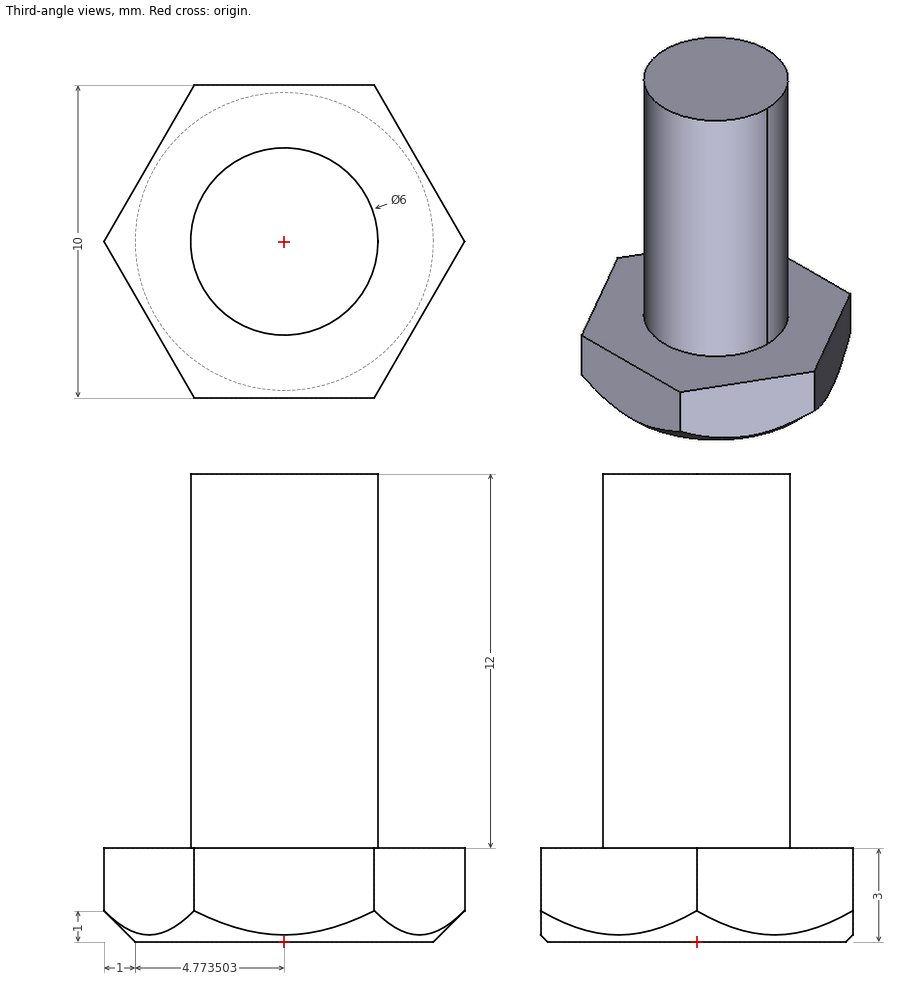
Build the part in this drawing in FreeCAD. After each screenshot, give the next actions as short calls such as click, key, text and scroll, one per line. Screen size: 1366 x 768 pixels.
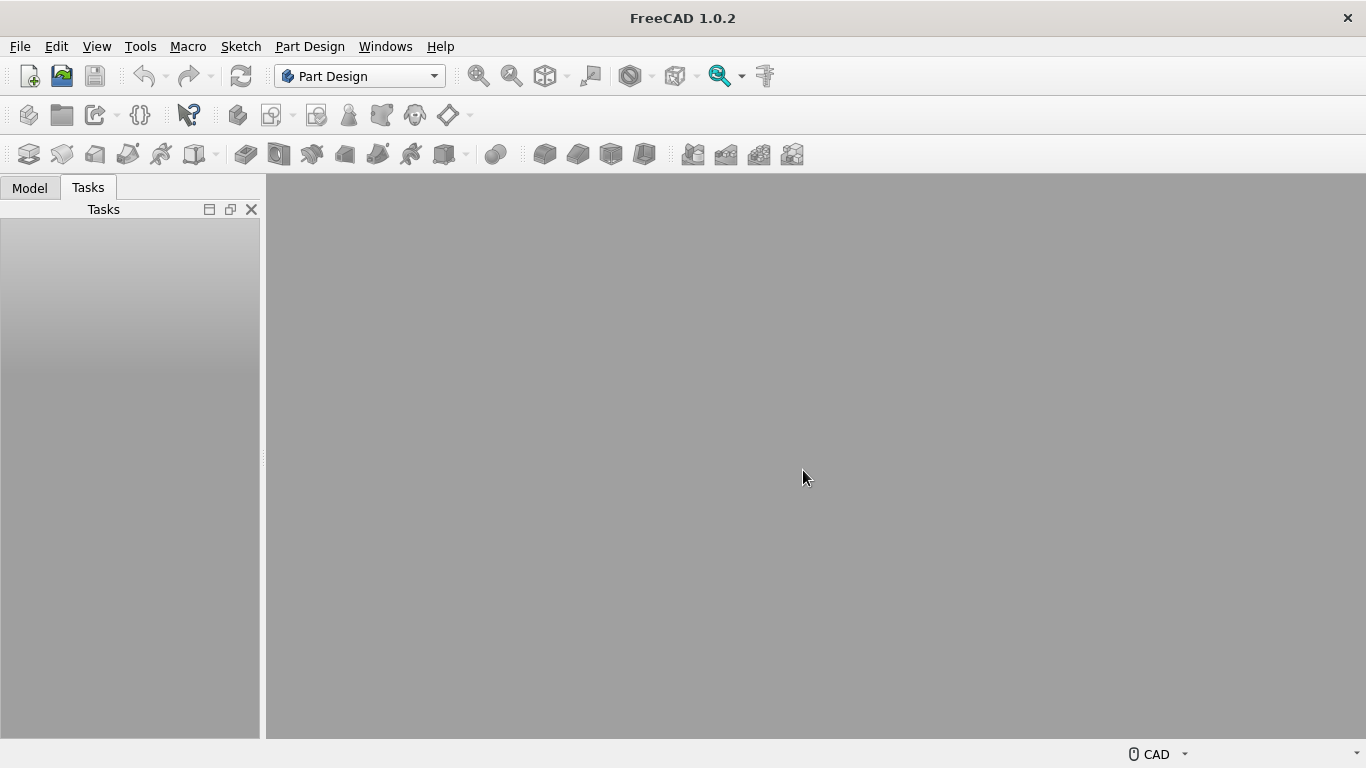
click(29, 76)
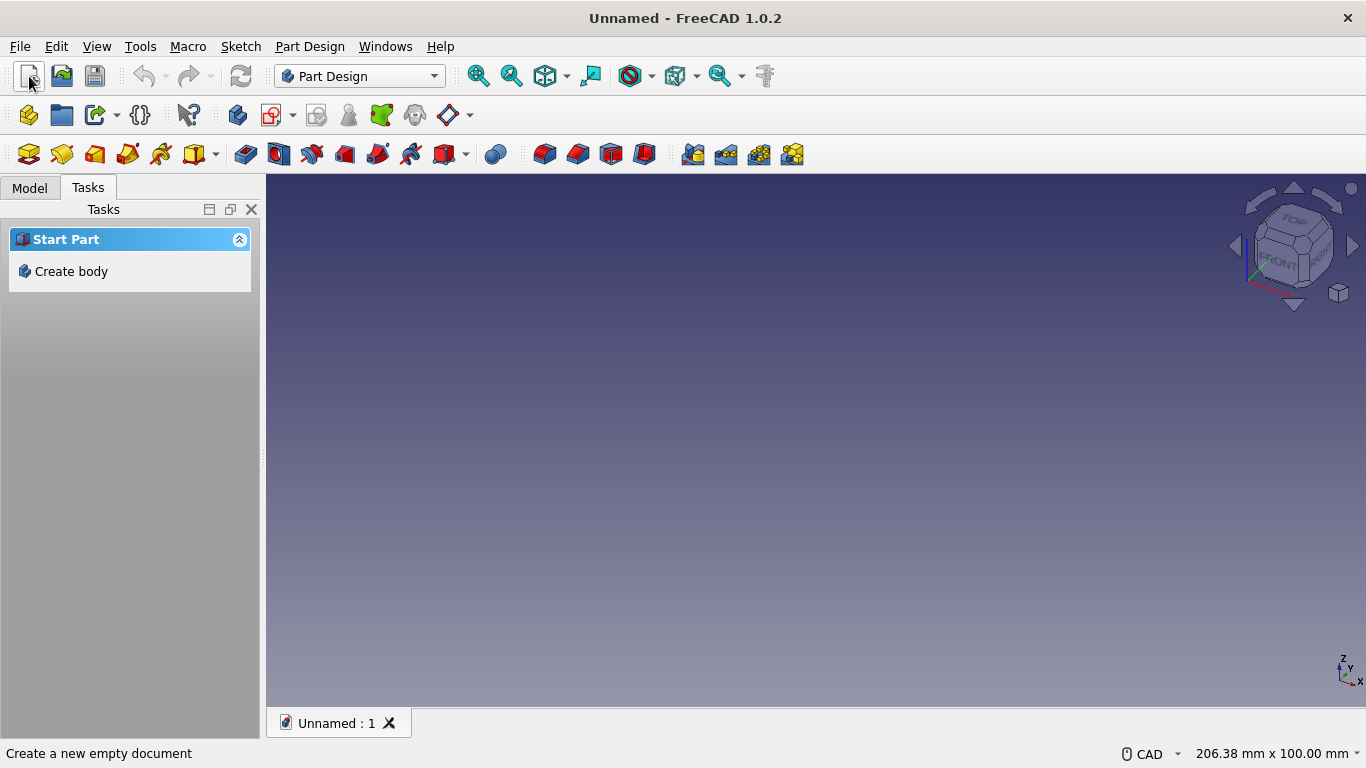
click(270, 116)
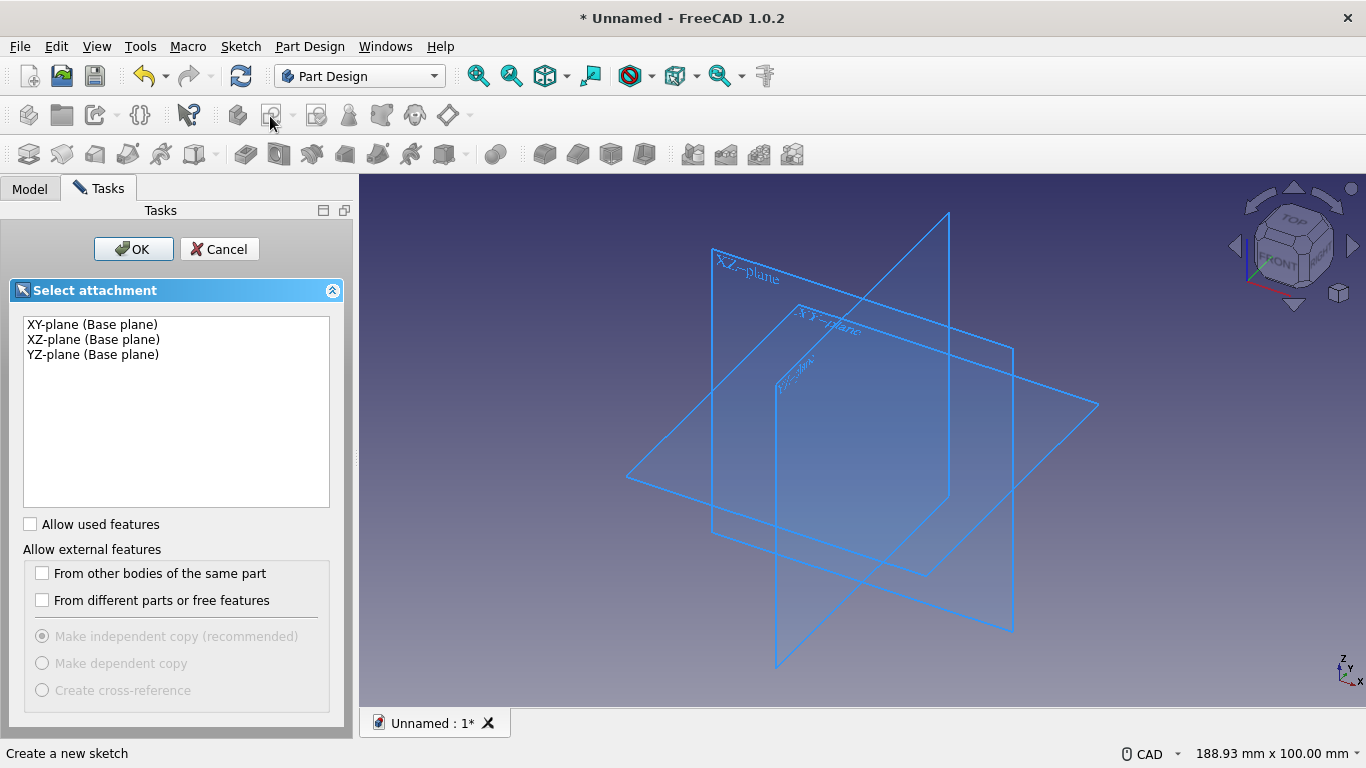
click(84, 324)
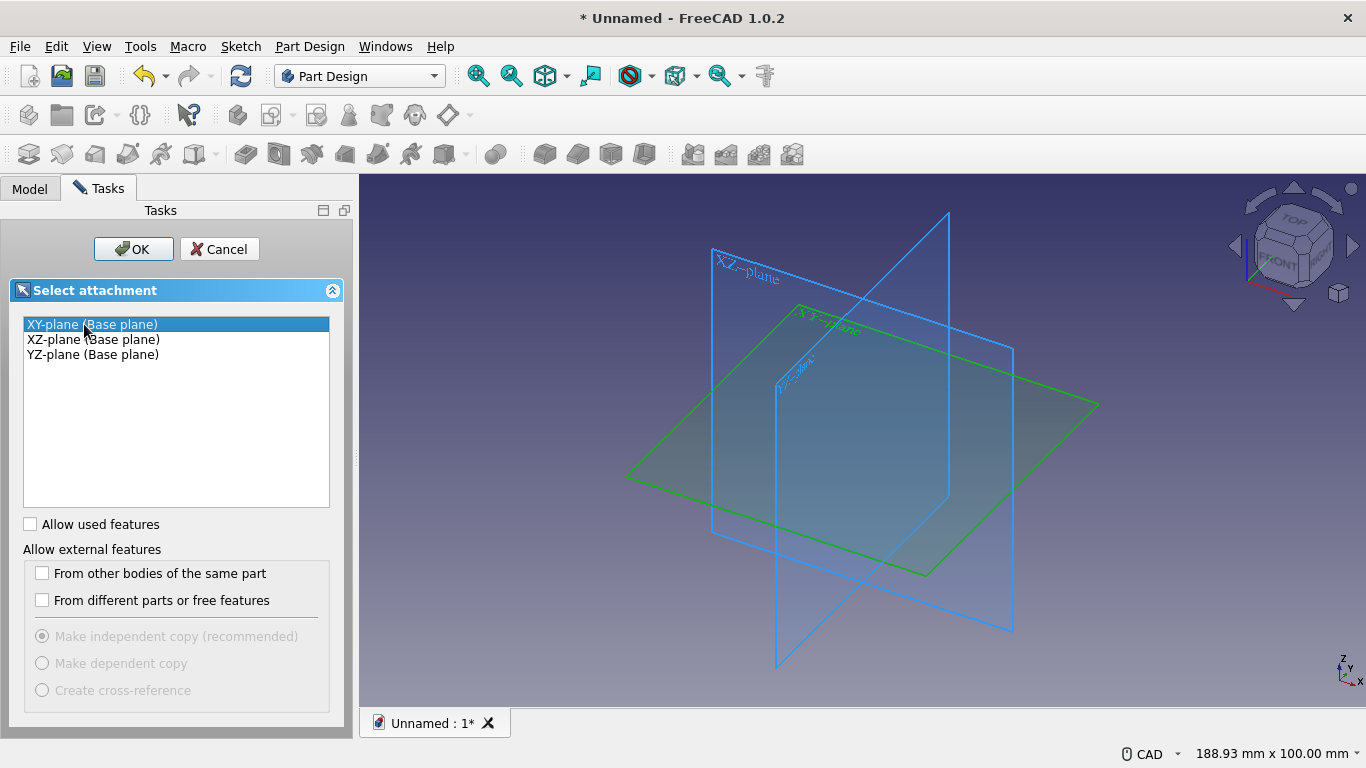
click(134, 249)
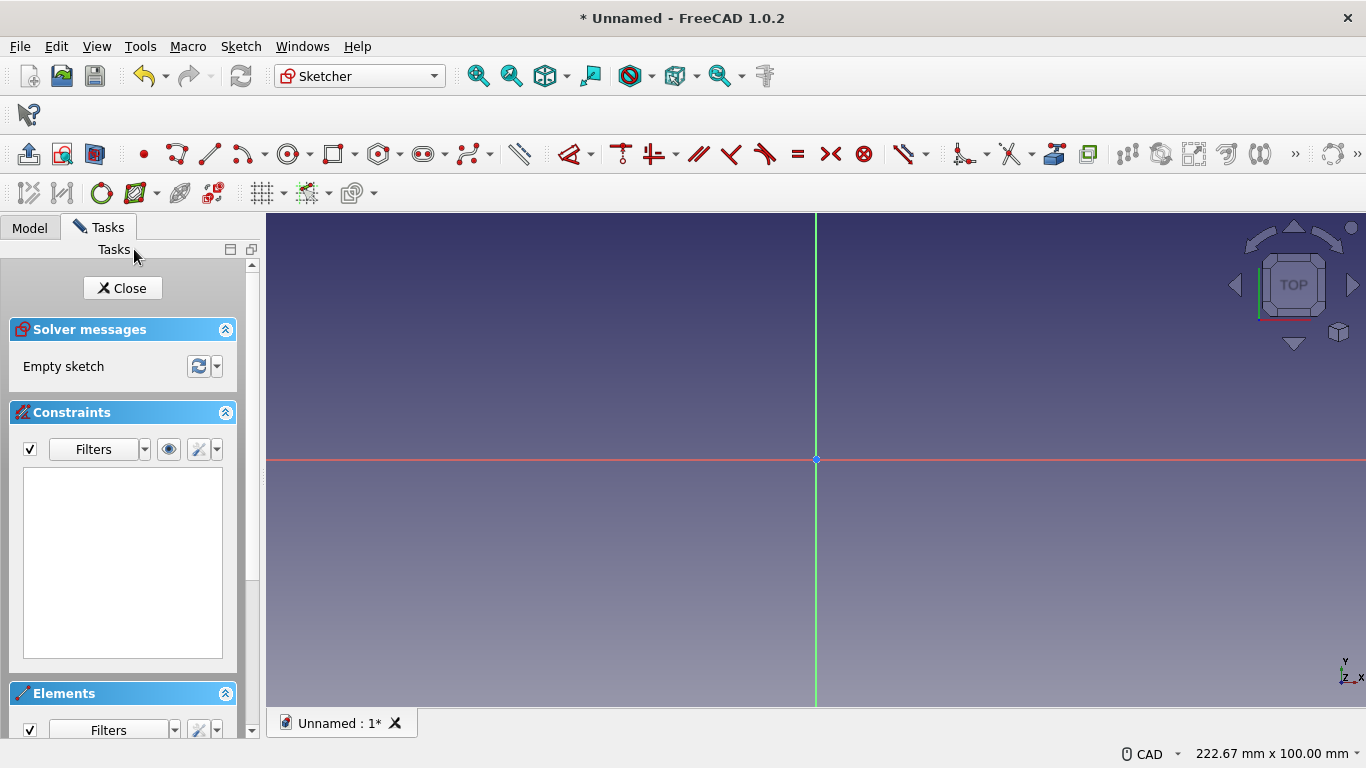
scroll(830, 460, up, 9)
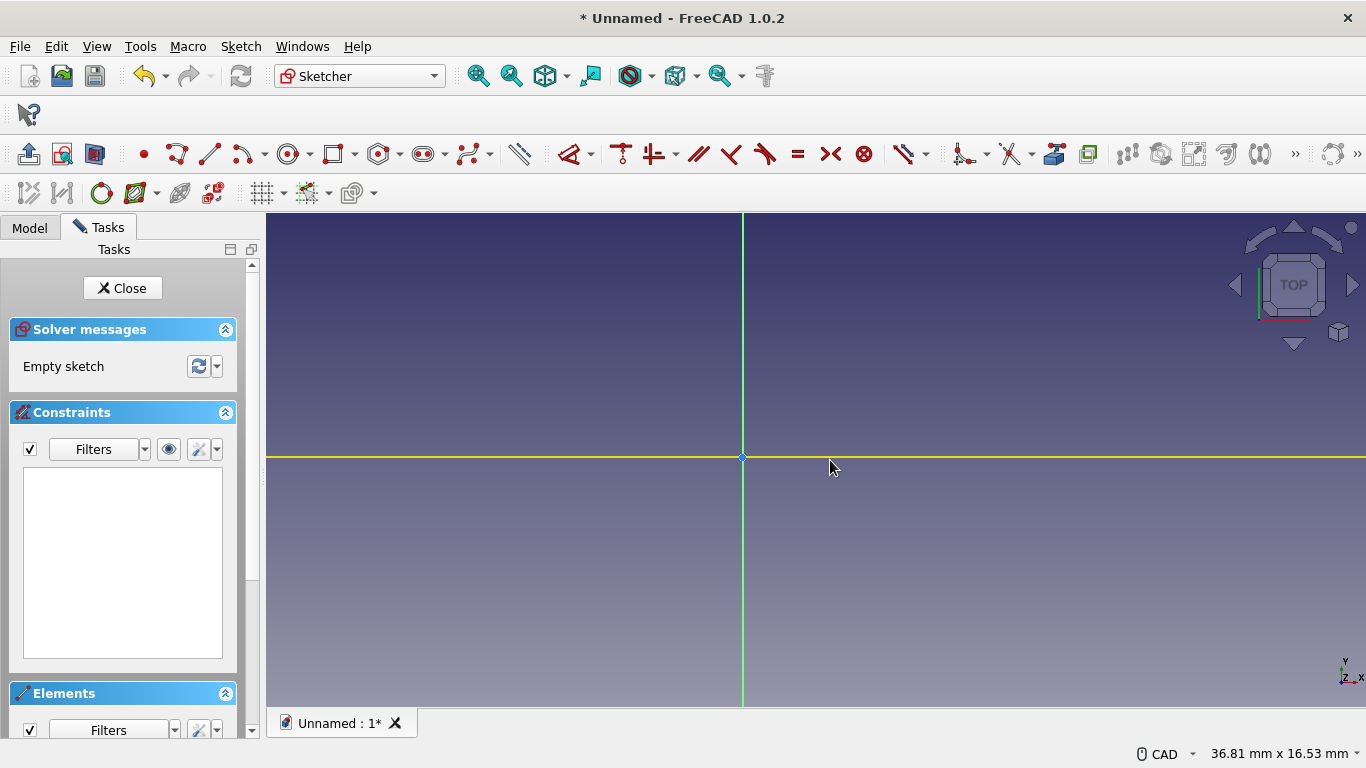
click(378, 154)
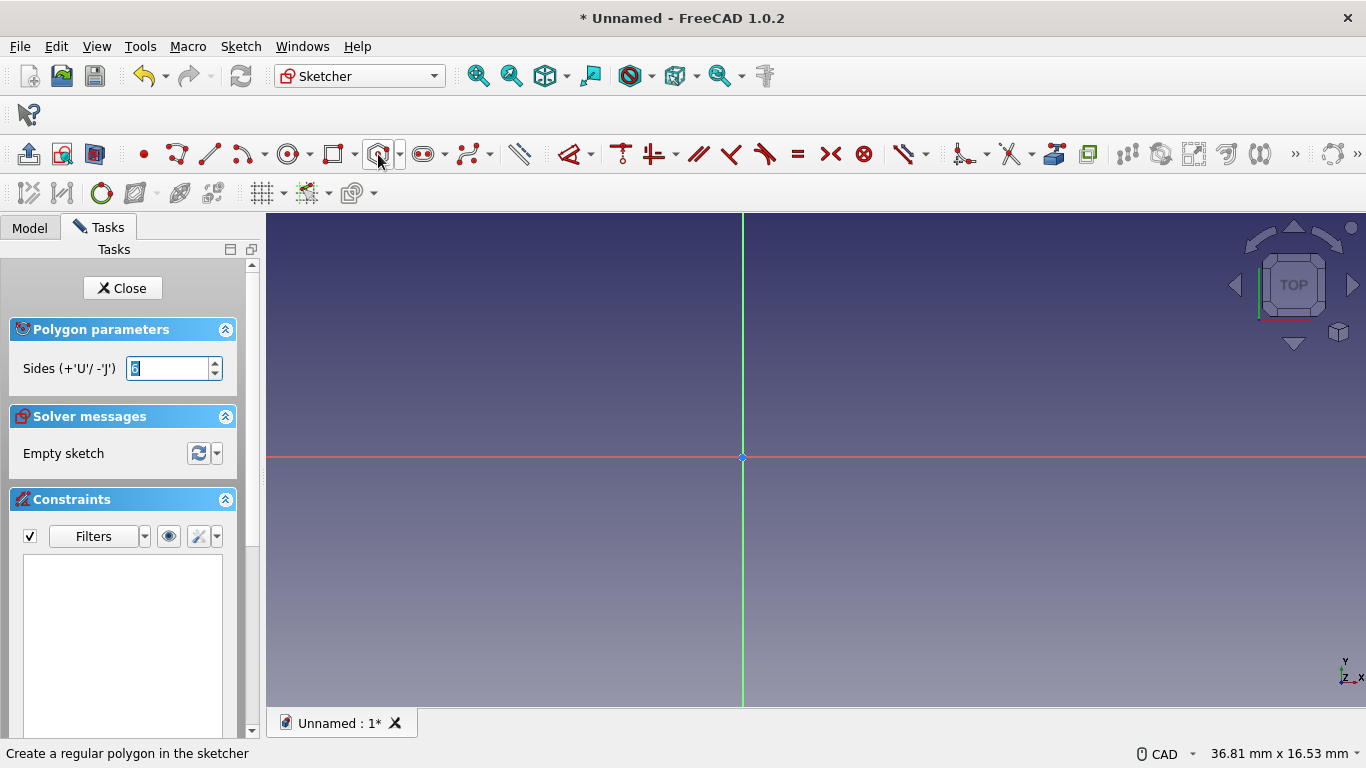
click(743, 457)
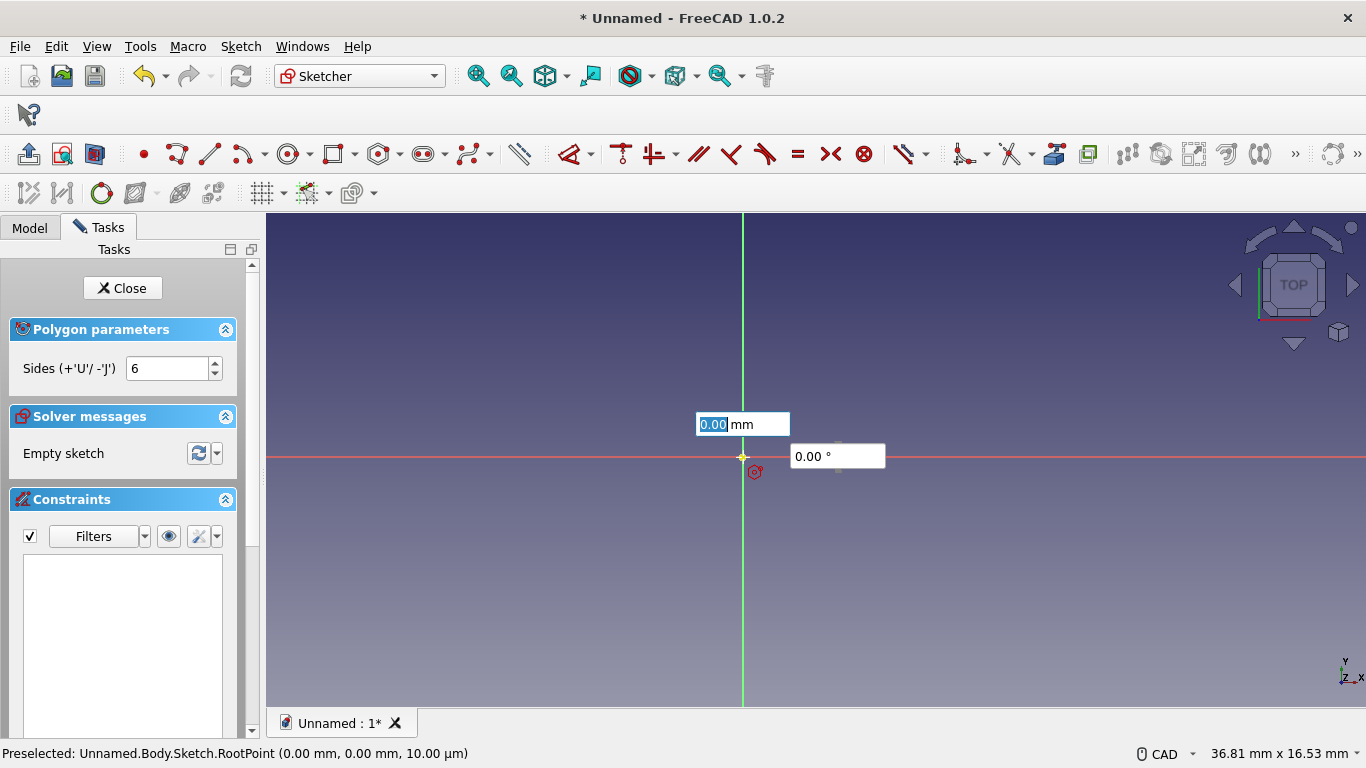
click(570, 457)
right_click(570, 457)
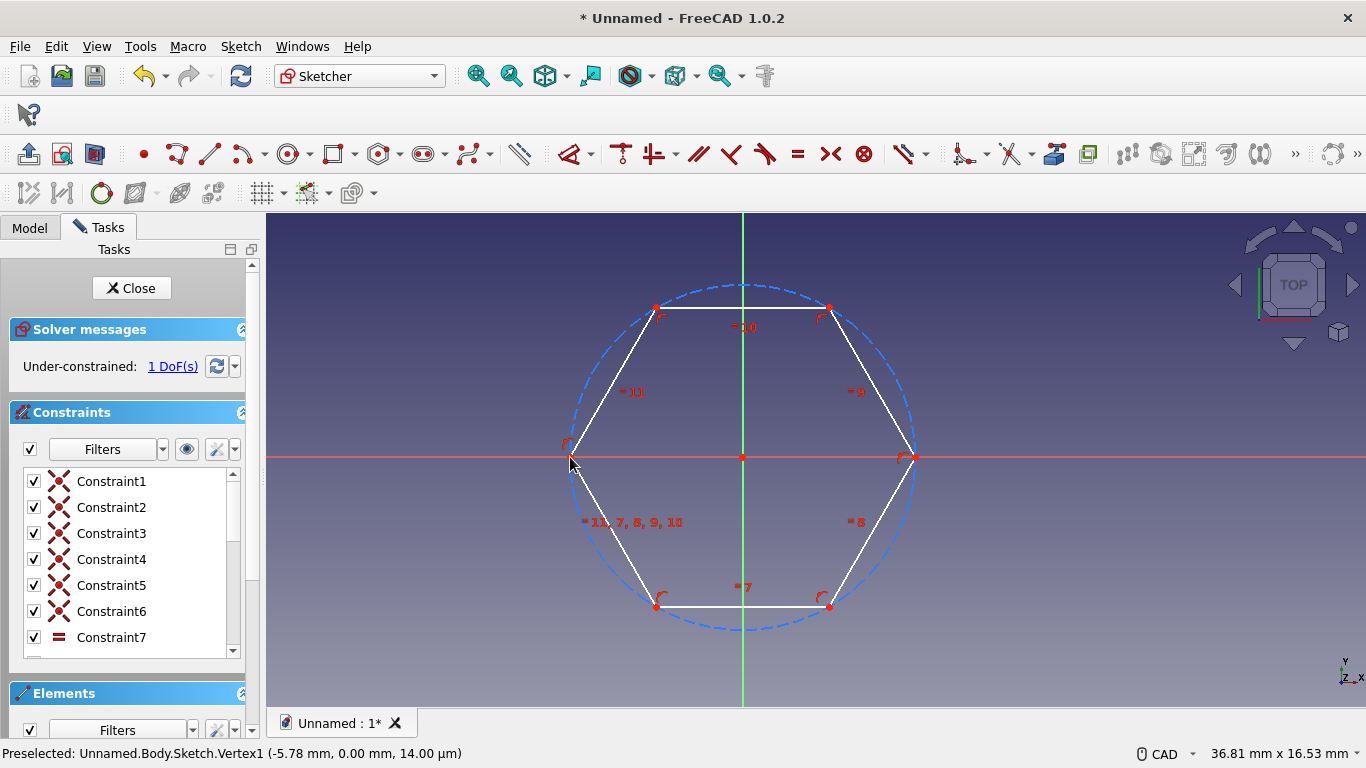
key(d)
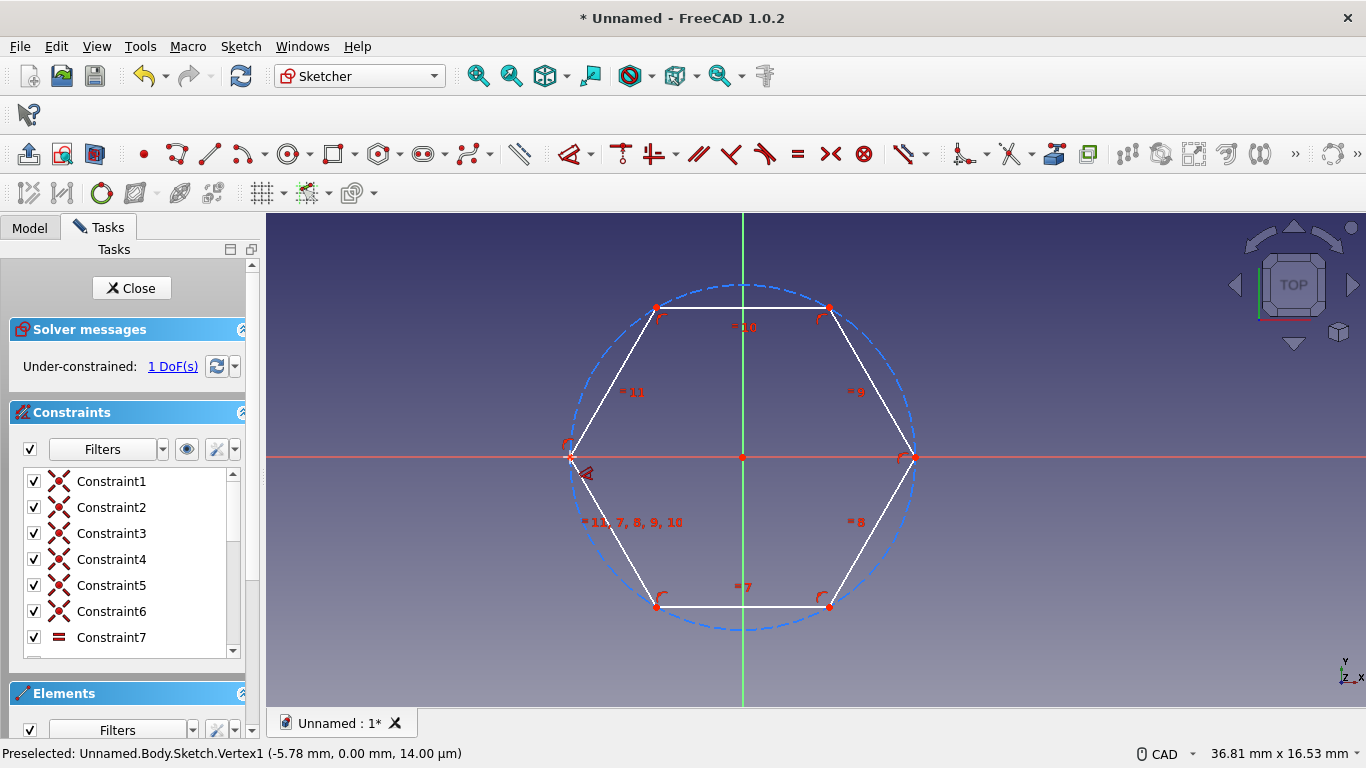
click(656, 607)